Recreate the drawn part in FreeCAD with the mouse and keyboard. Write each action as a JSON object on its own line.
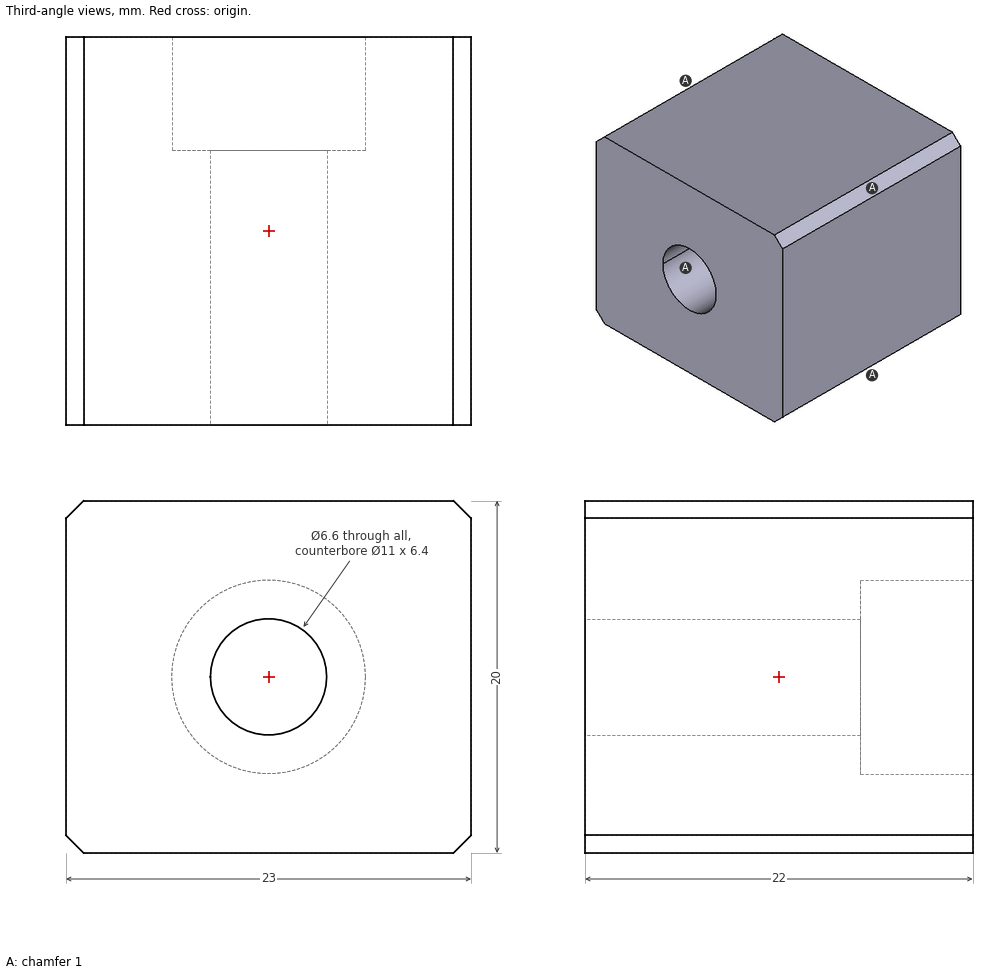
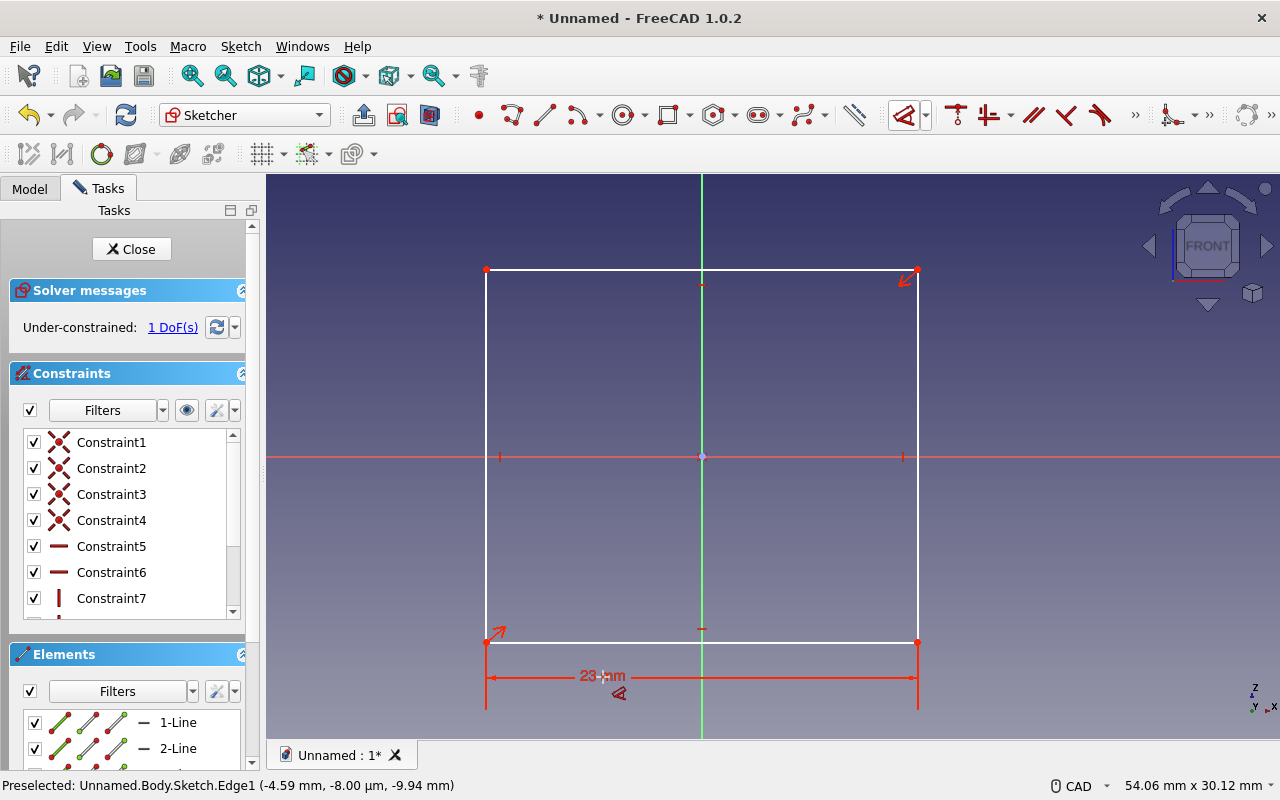
{"action": "left_click", "coordinate": [918, 531]}
{"action": "left_click", "coordinate": [952, 371]}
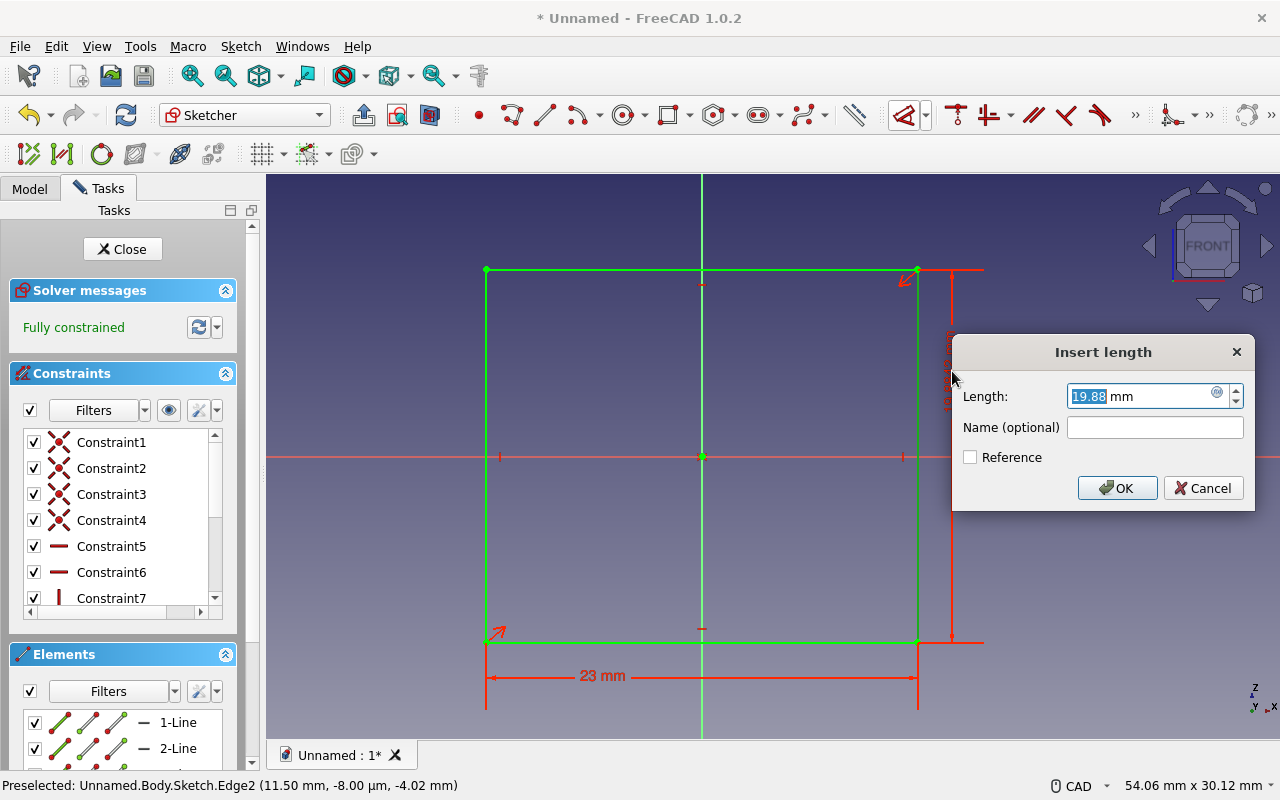
{"action": "type", "text": "20"}
{"action": "key", "text": "Return"}
{"action": "key", "text": "Escape"}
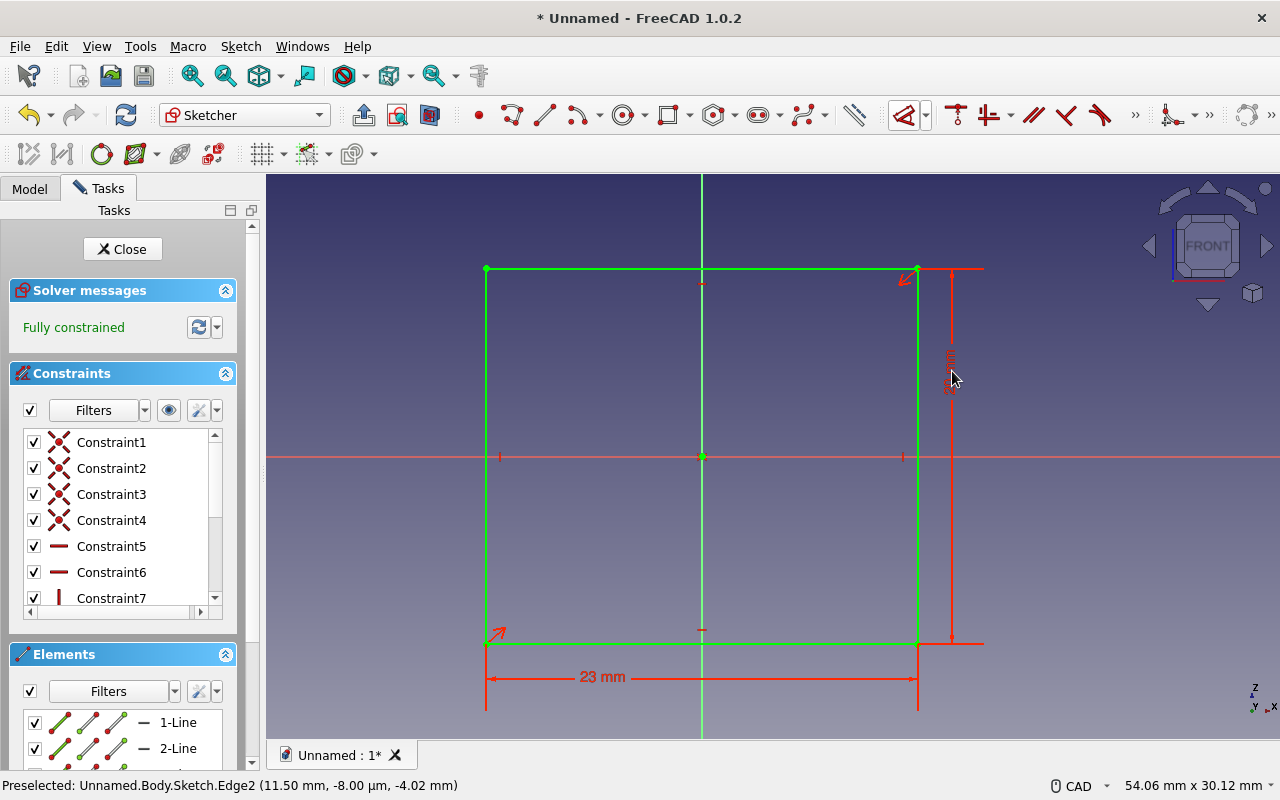
{"action": "left_click", "coordinate": [123, 249]}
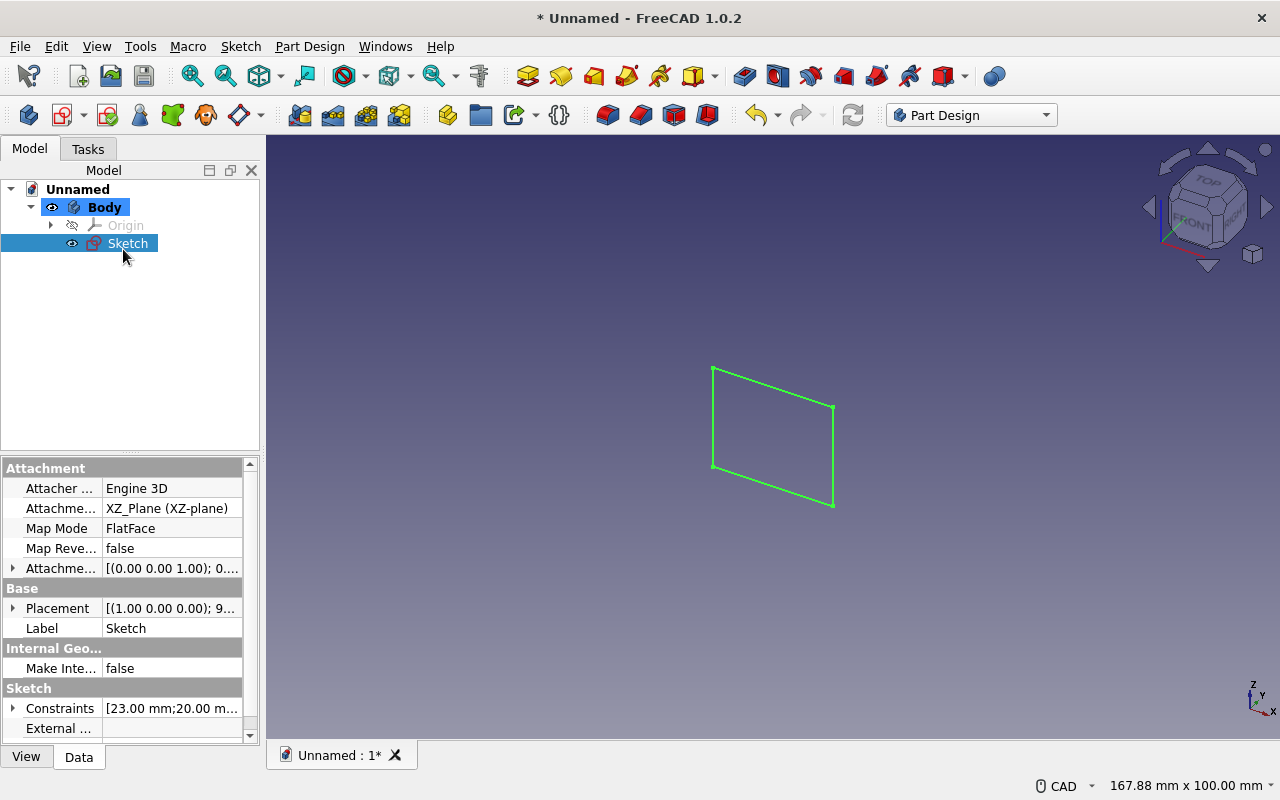
{"action": "left_click", "coordinate": [528, 76]}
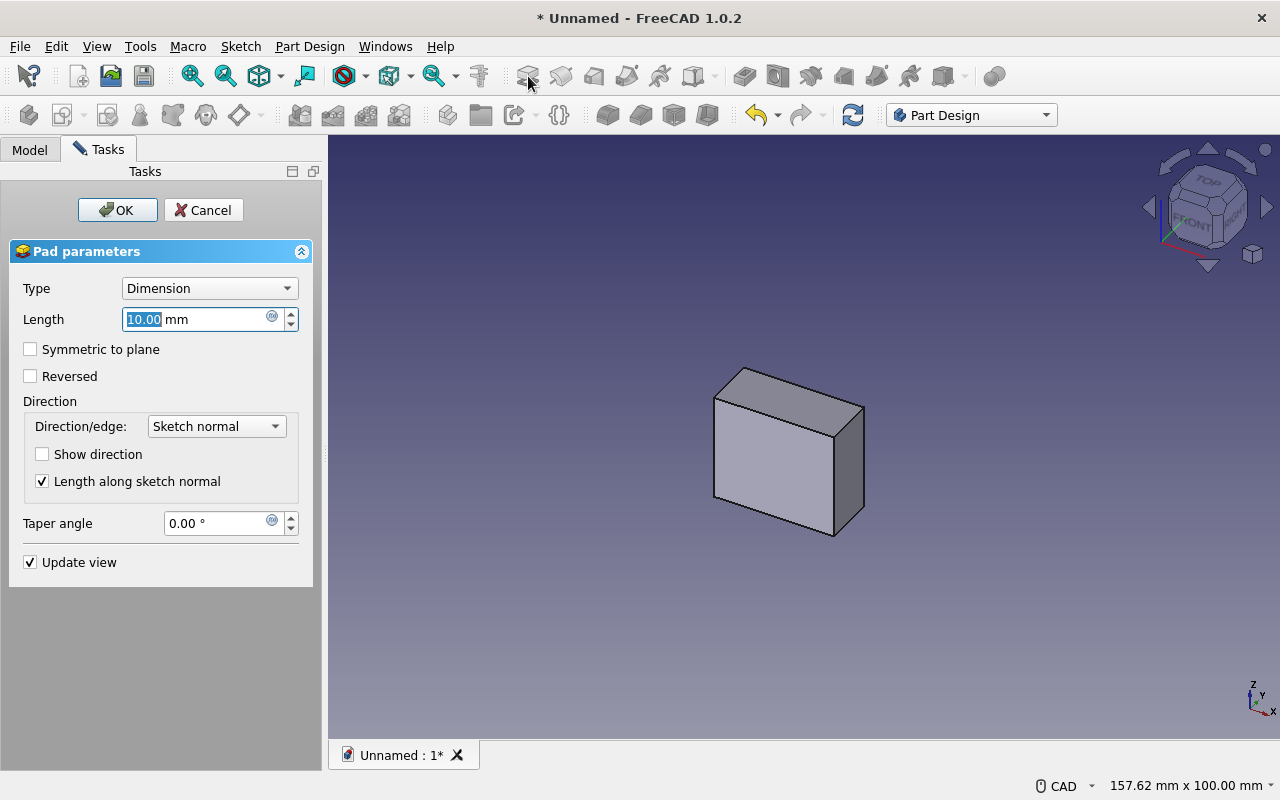
{"action": "type", "text": "22"}
{"action": "key", "text": "Tab"}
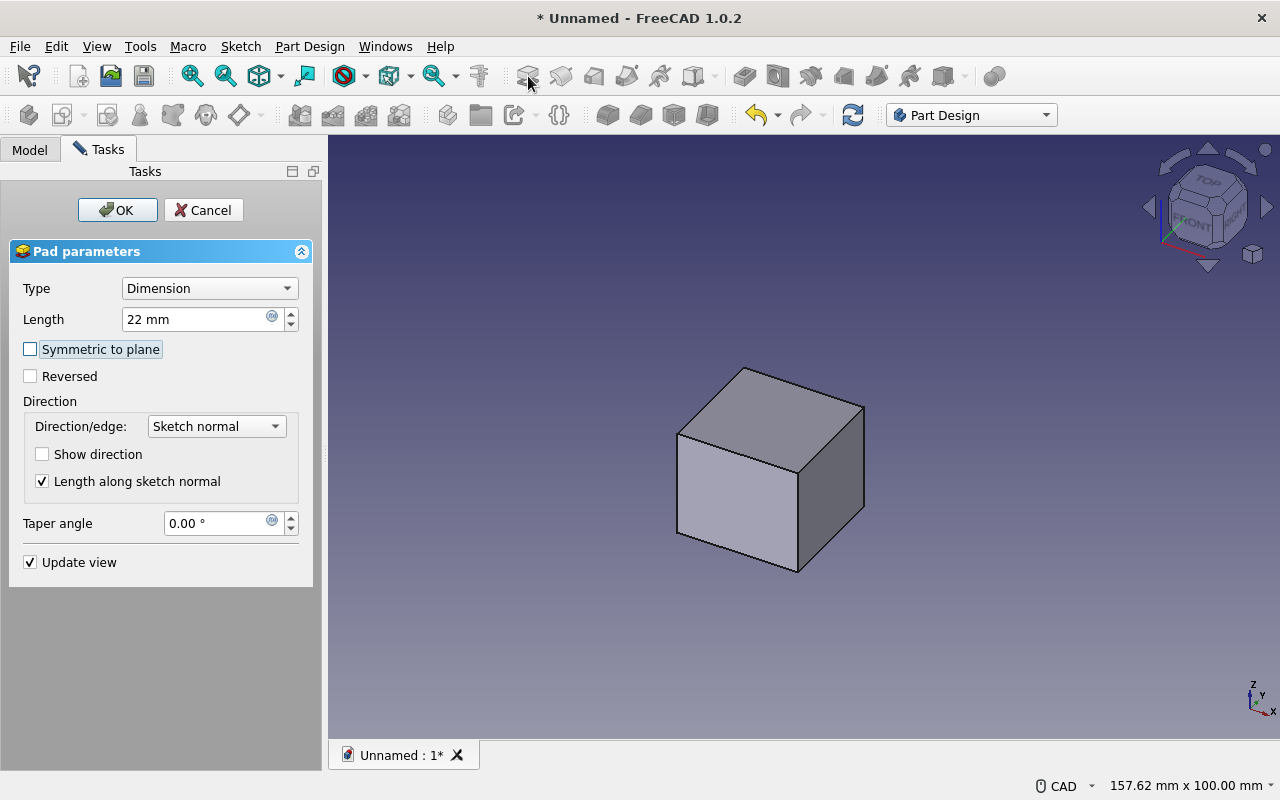
{"action": "left_click", "coordinate": [31, 349]}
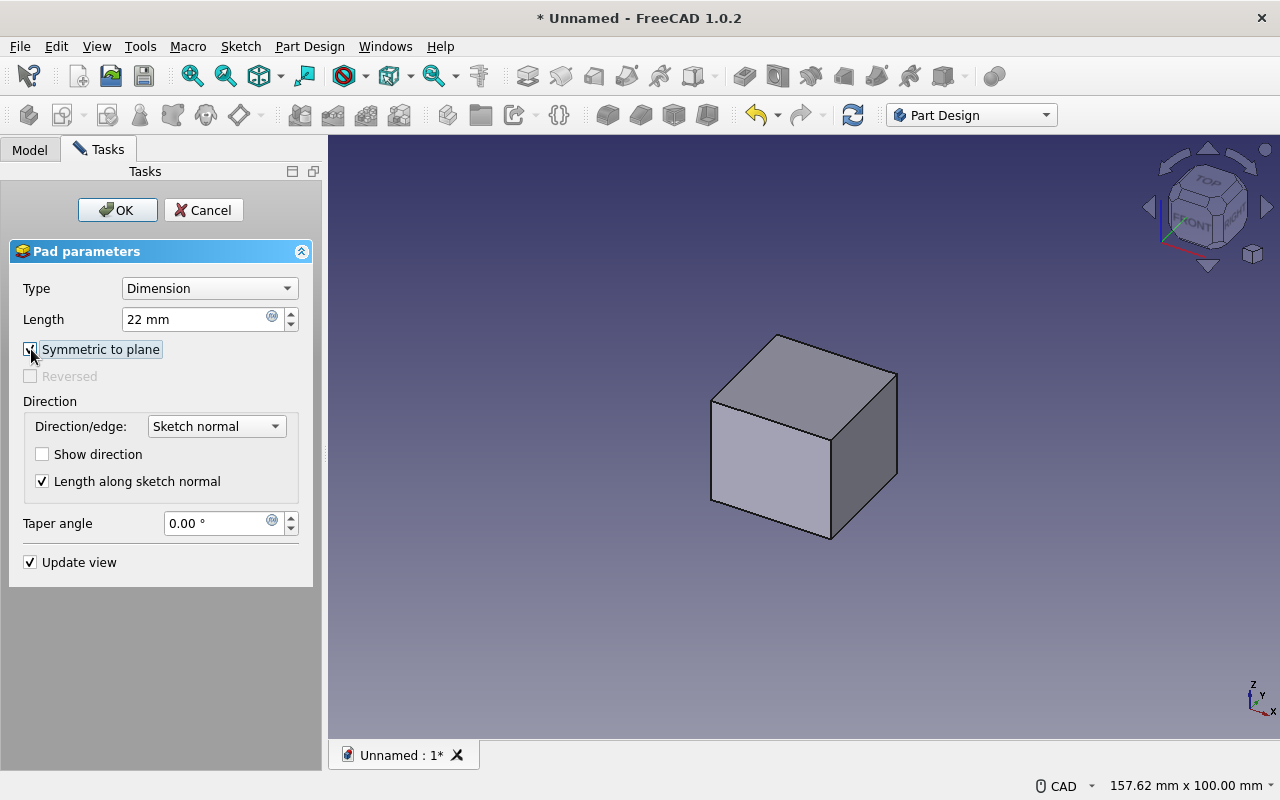
{"action": "left_click", "coordinate": [118, 210]}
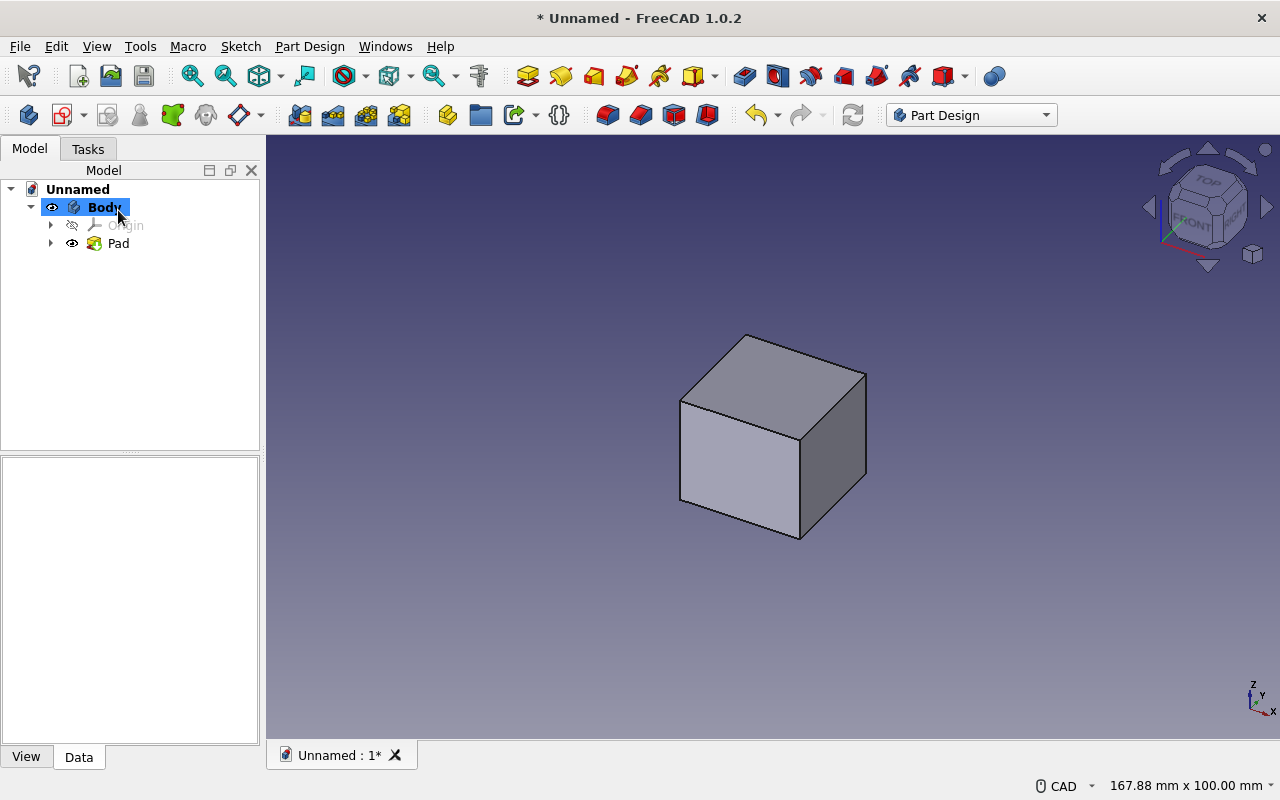
{"action": "left_click", "coordinate": [193, 76]}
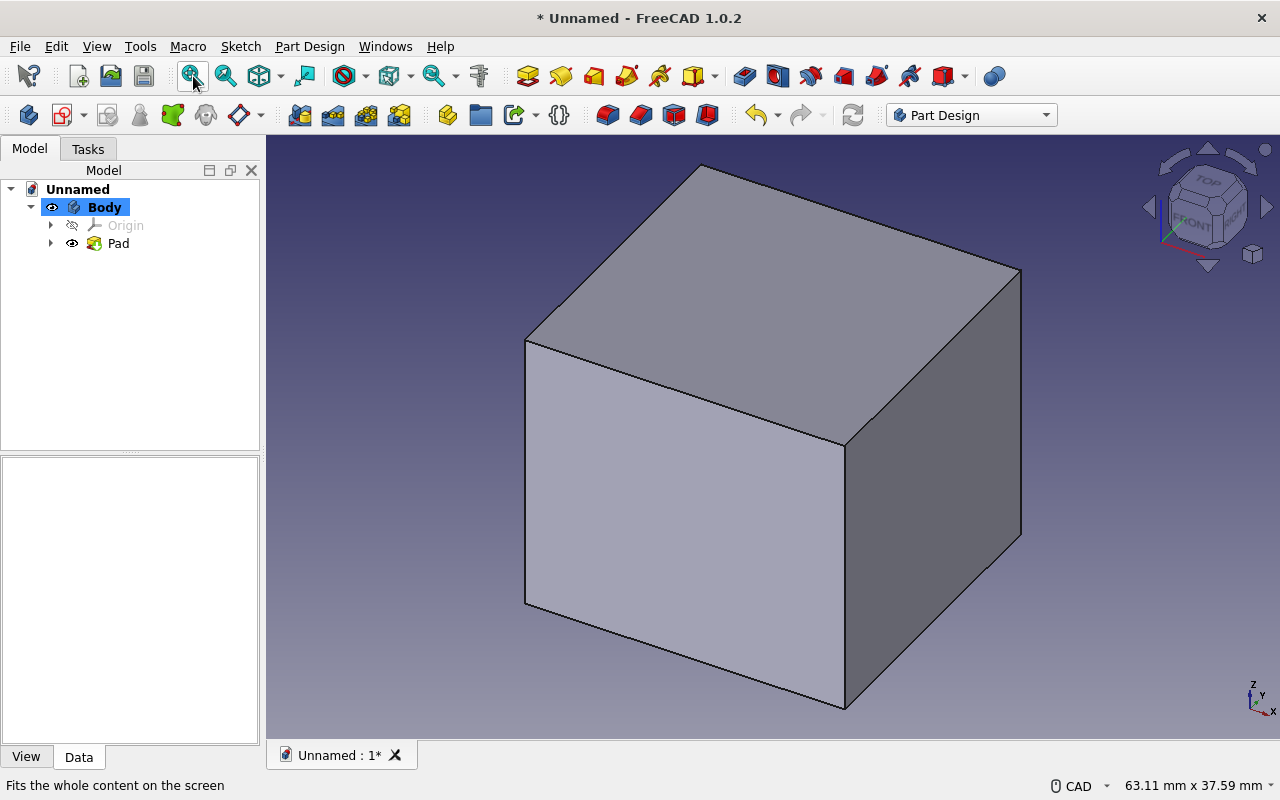
{"action": "key", "text": "4"}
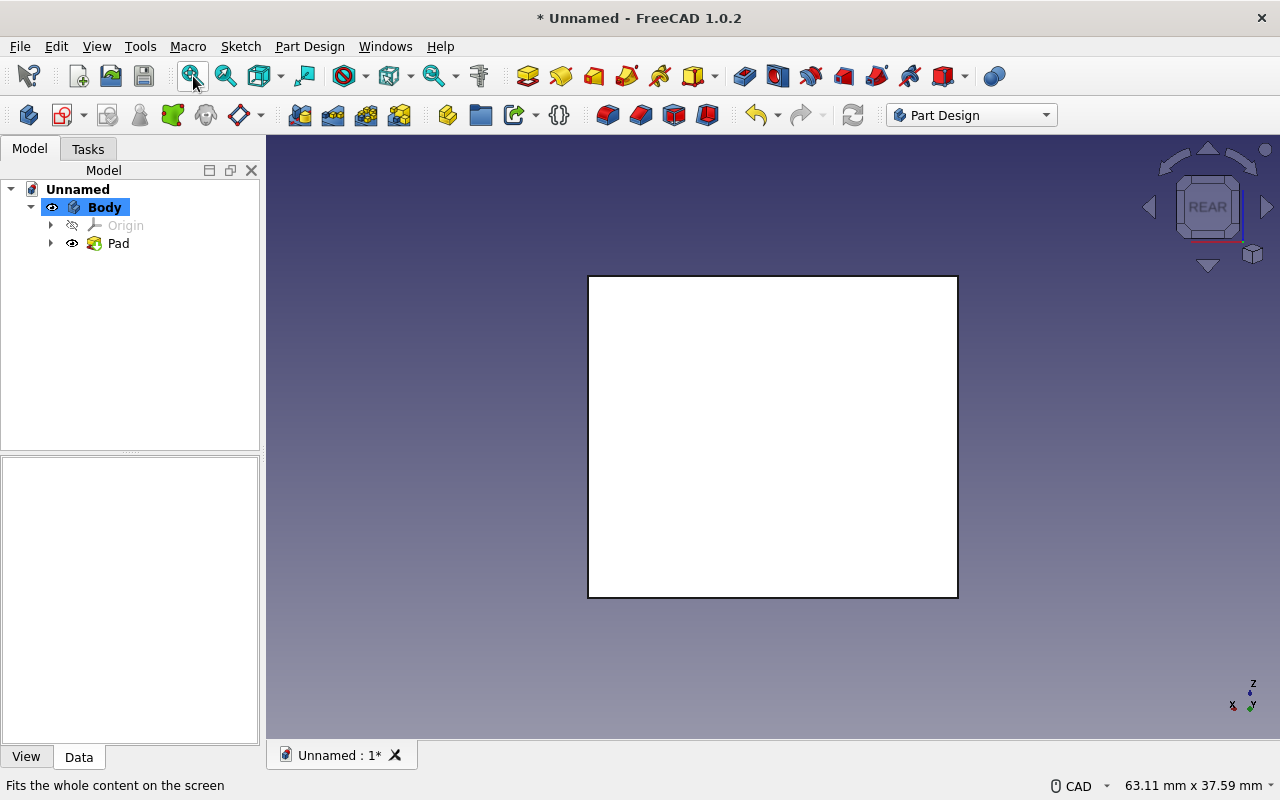
{"action": "left_click", "coordinate": [773, 436]}